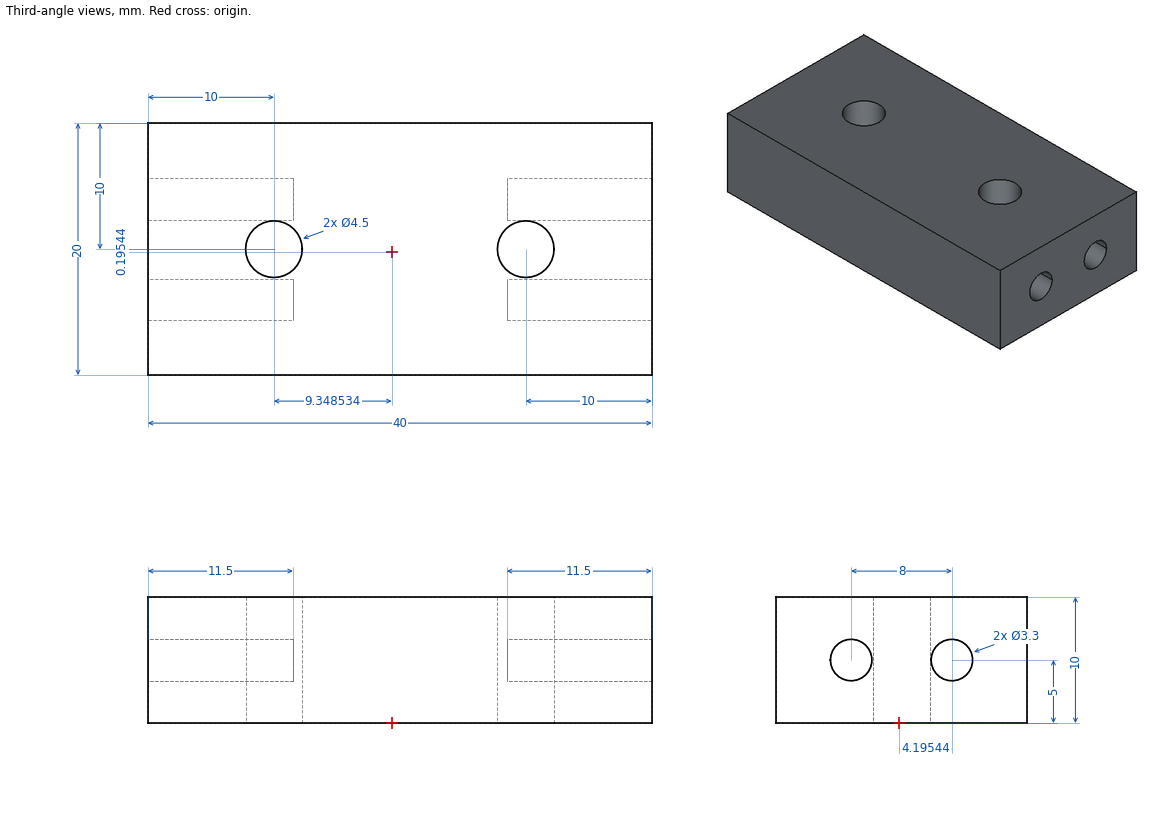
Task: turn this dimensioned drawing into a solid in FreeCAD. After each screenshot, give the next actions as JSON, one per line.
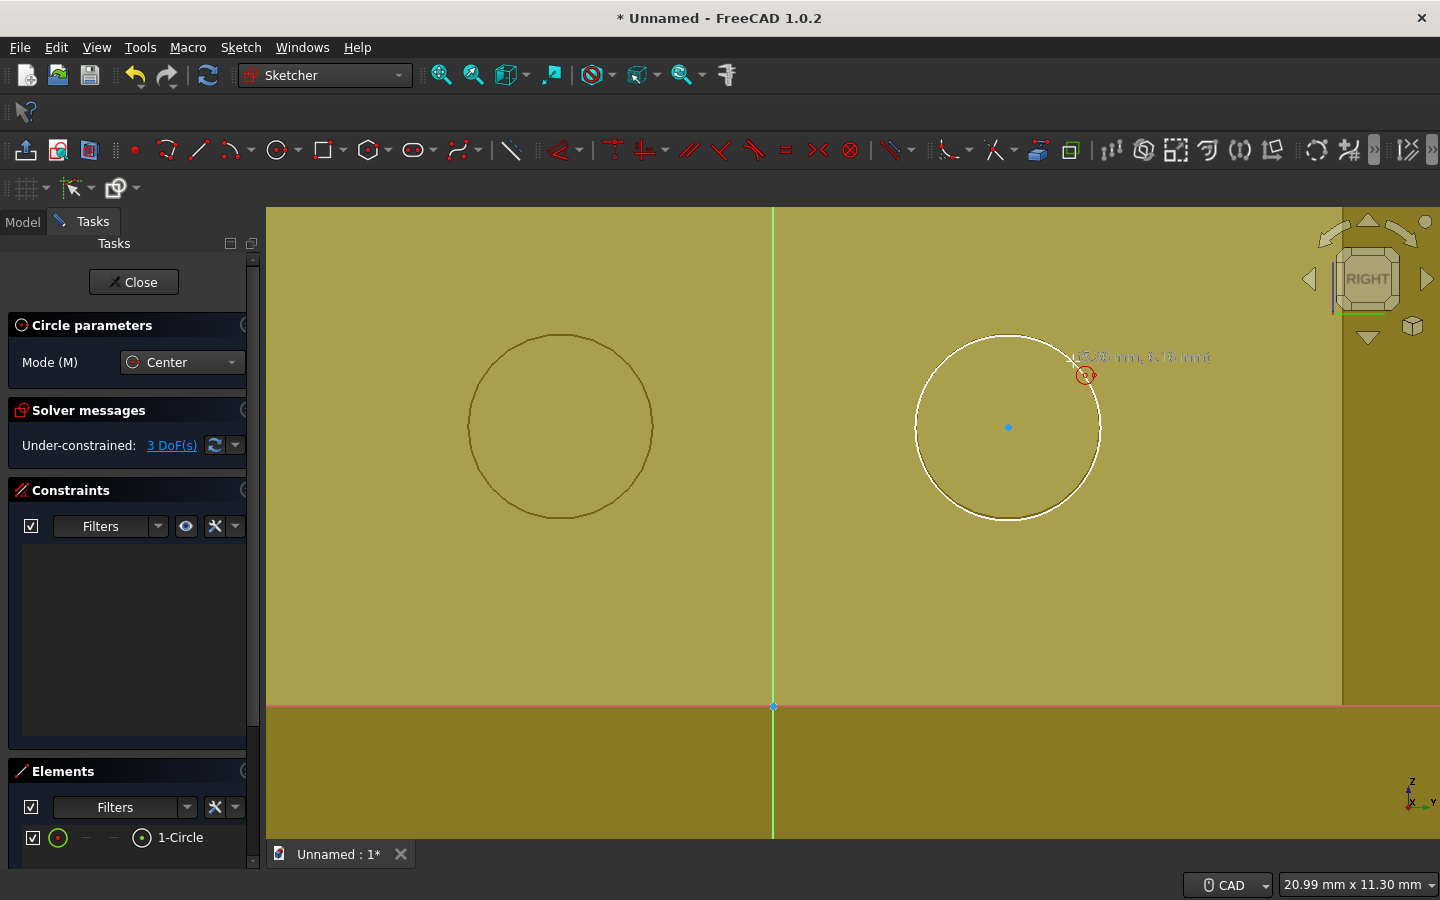
{"action": "left_click", "coordinate": [560, 427]}
{"action": "left_click", "coordinate": [626, 361]}
{"action": "key", "text": "Escape"}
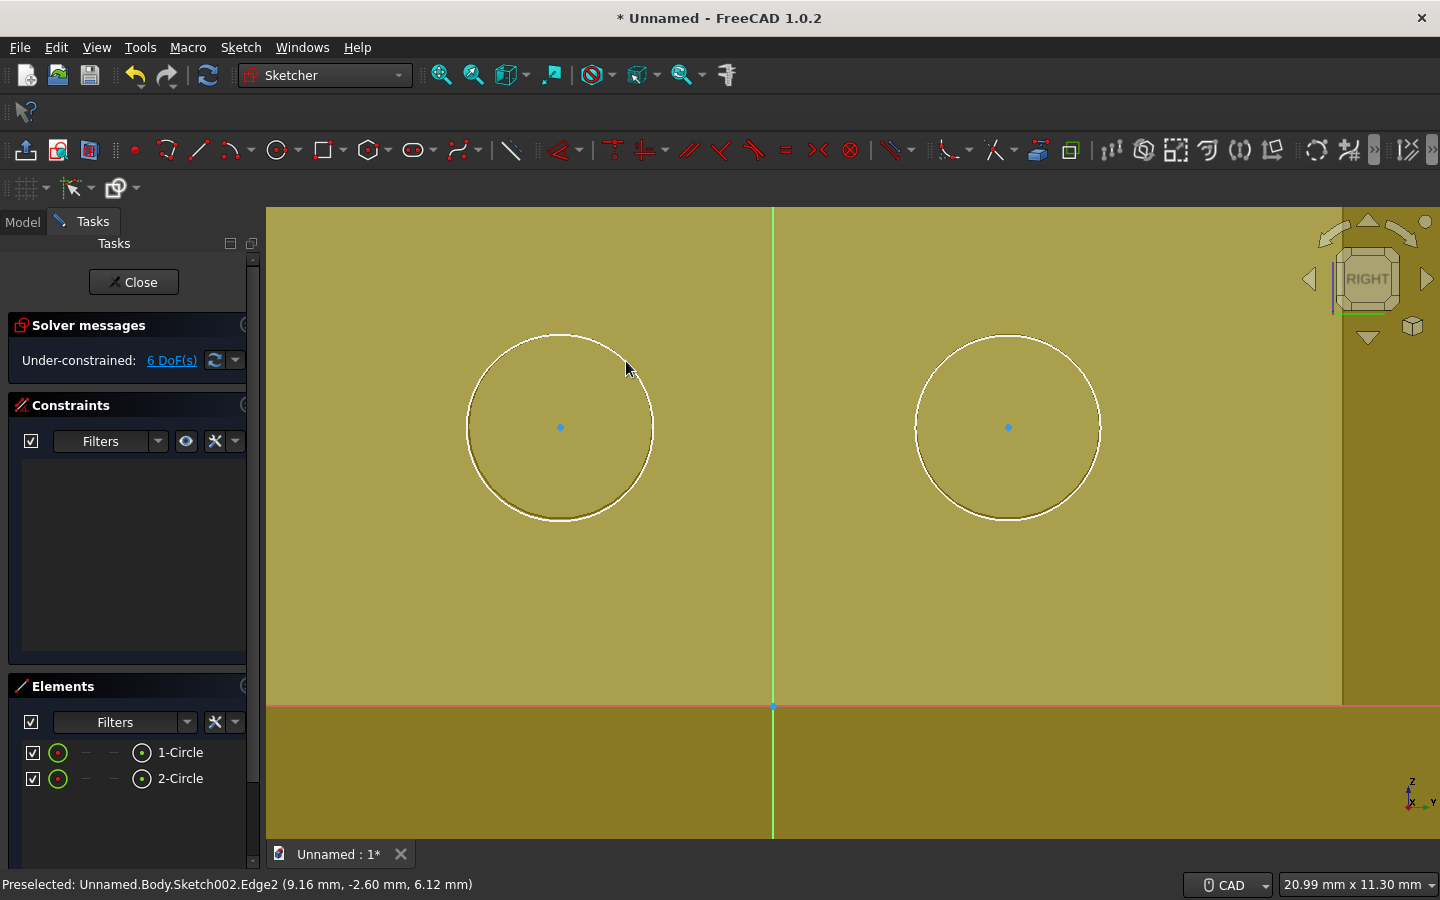
{"action": "left_click", "coordinate": [1073, 362]}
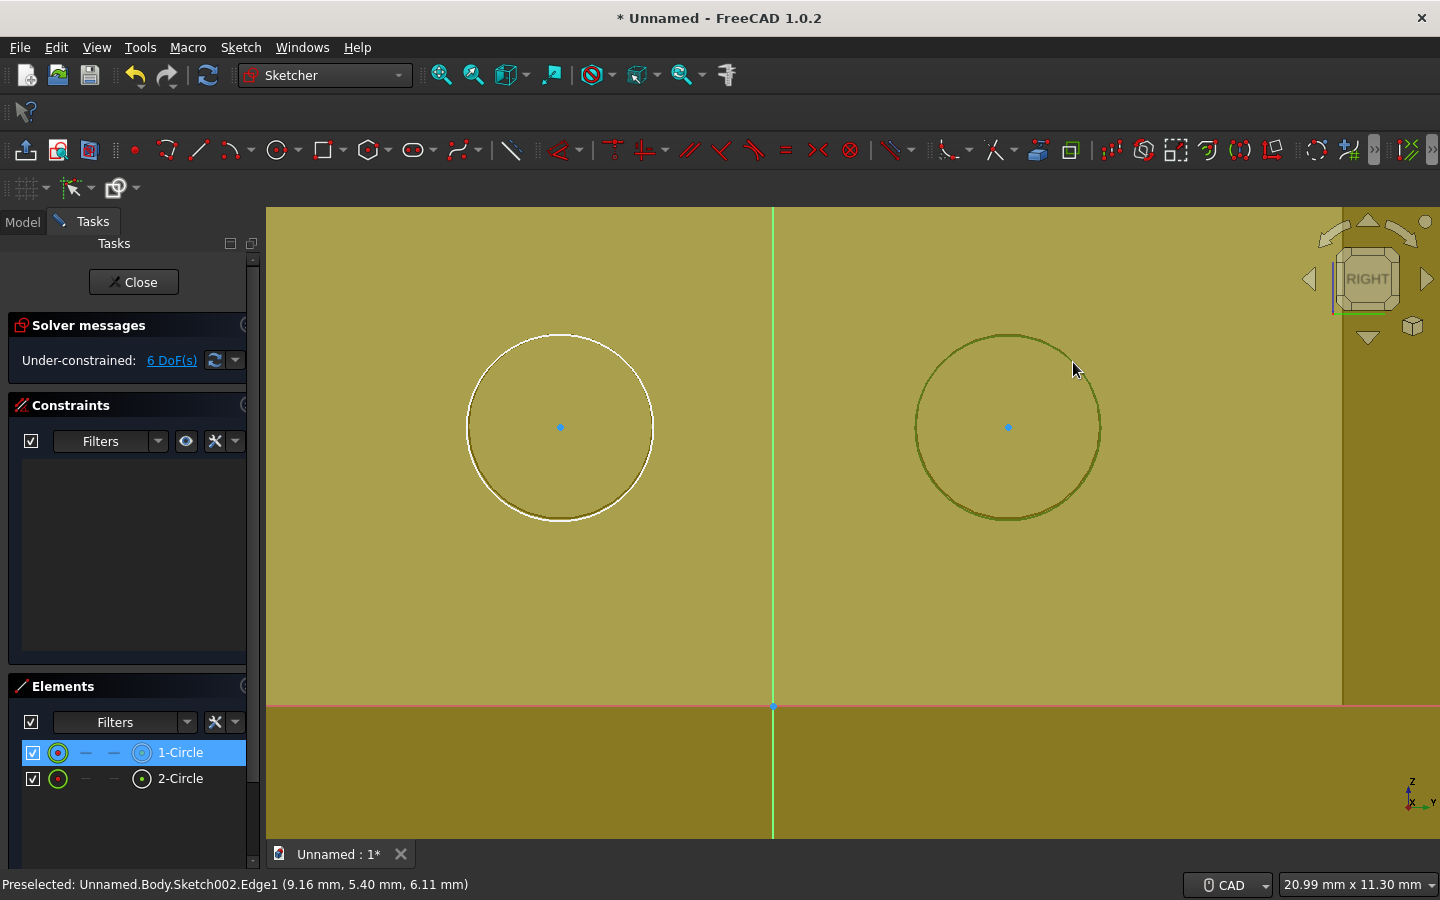
{"action": "left_click", "coordinate": [626, 362]}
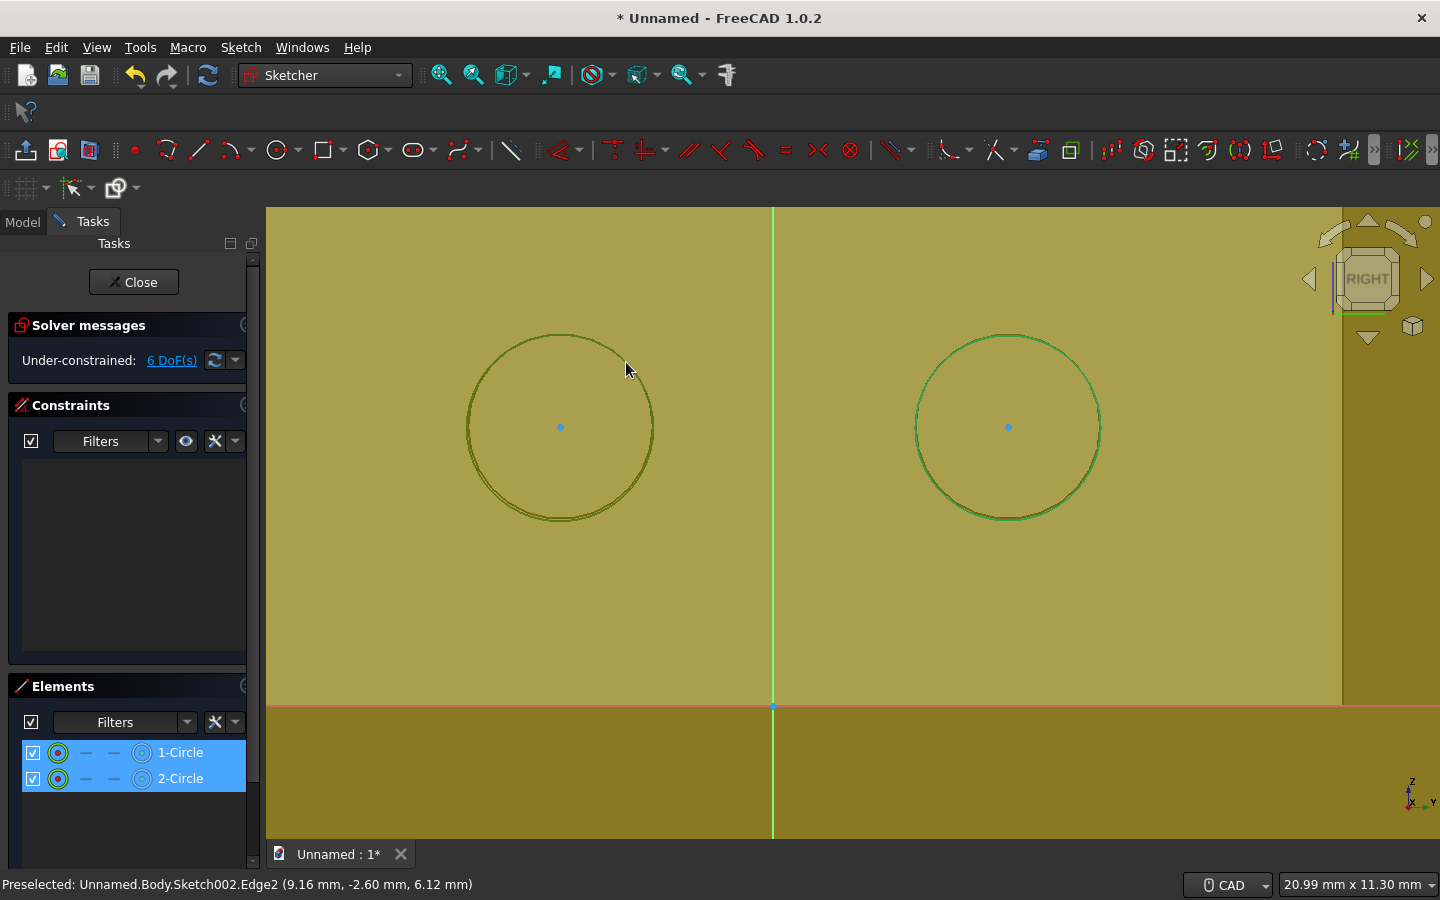
{"action": "key", "text": "e"}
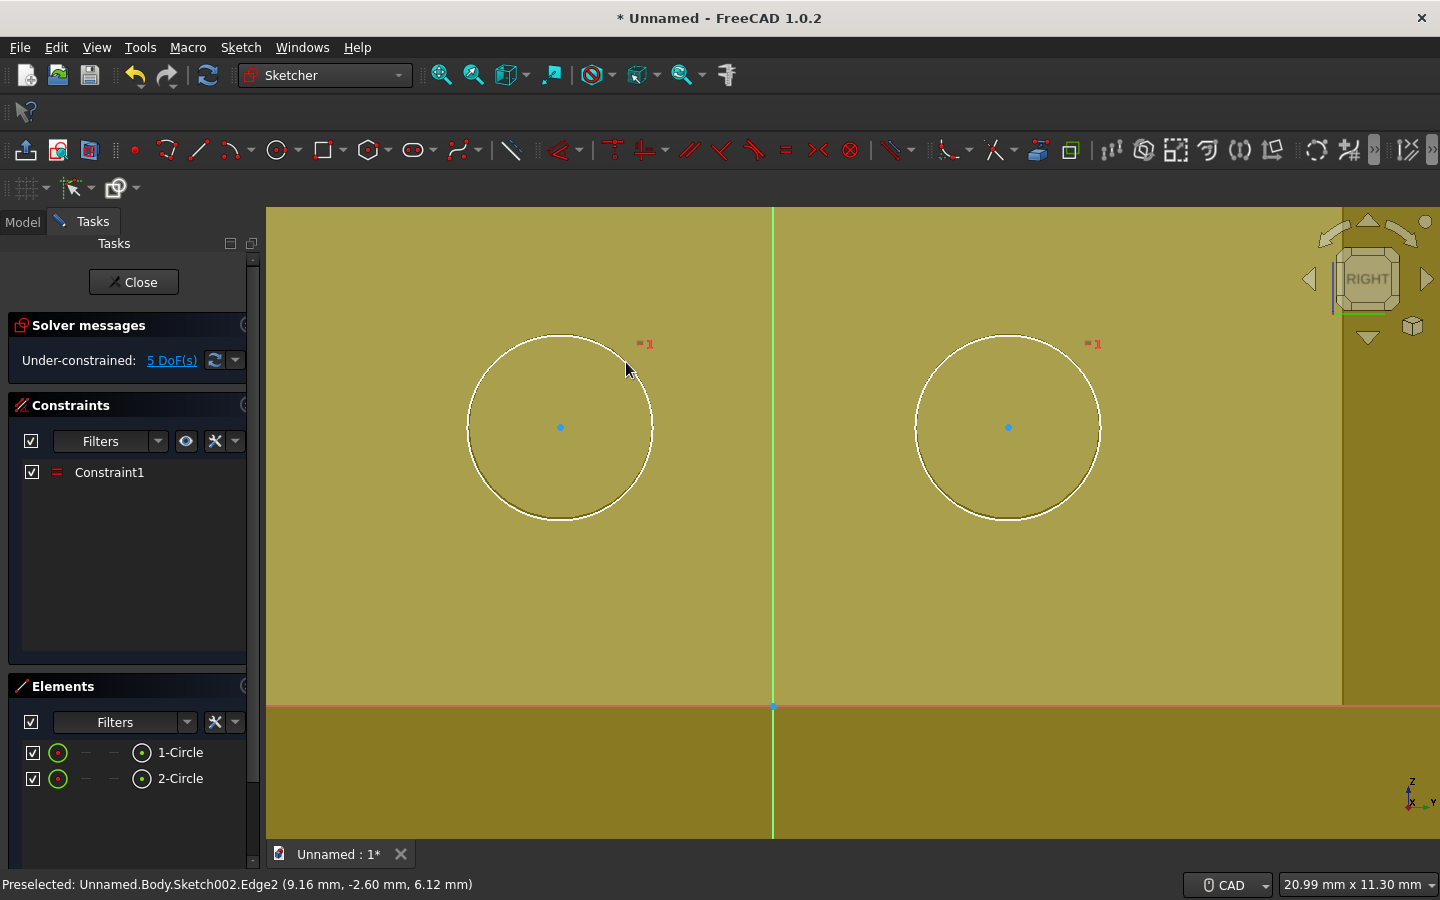
{"action": "left_click", "coordinate": [1008, 428]}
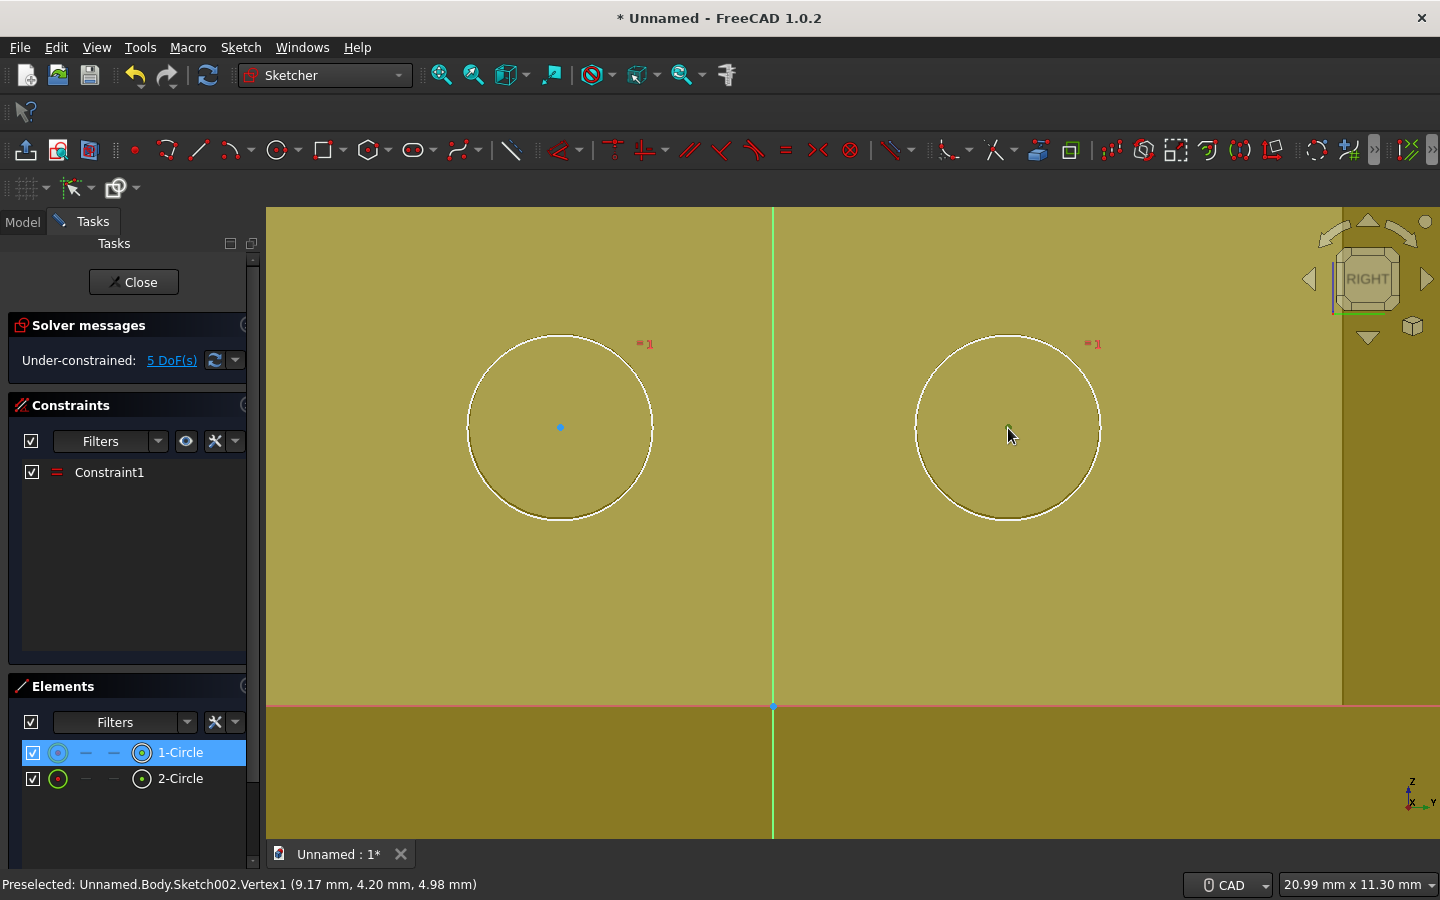
{"action": "left_click", "coordinate": [560, 428]}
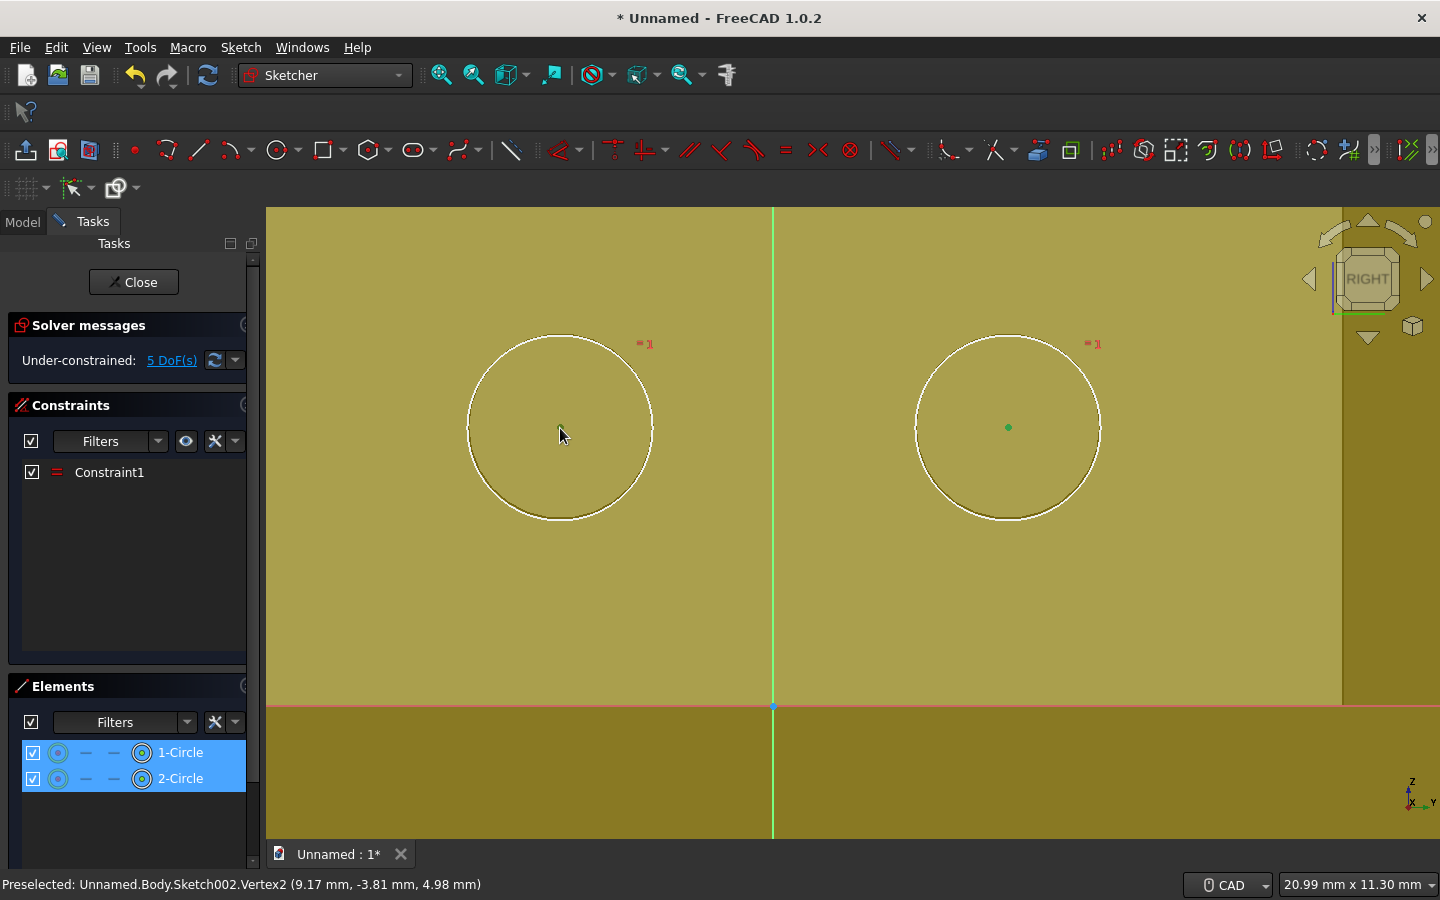
{"action": "key", "text": "h"}